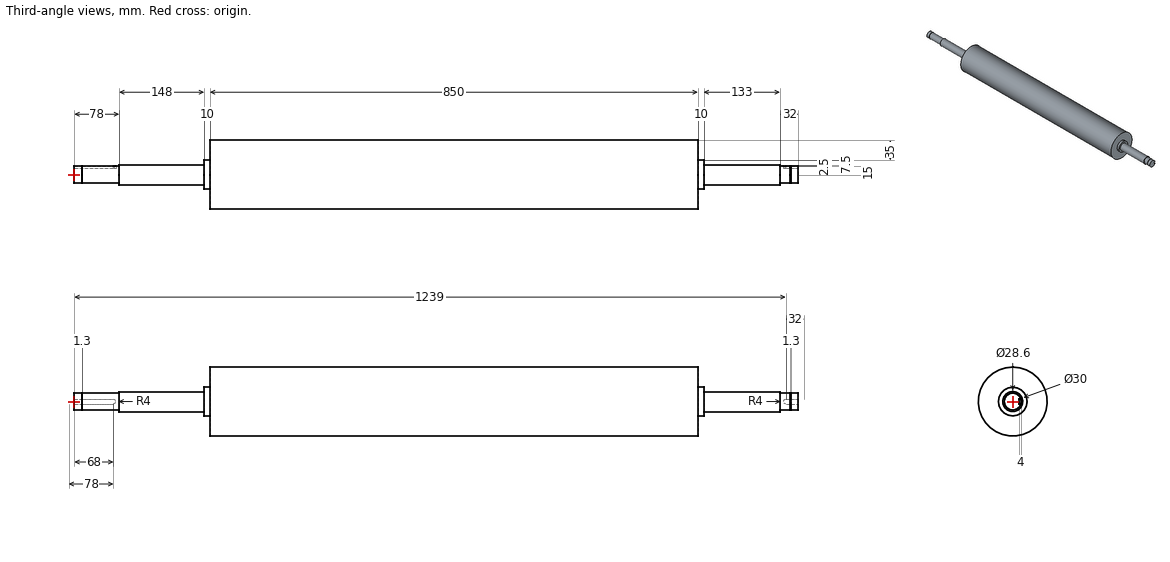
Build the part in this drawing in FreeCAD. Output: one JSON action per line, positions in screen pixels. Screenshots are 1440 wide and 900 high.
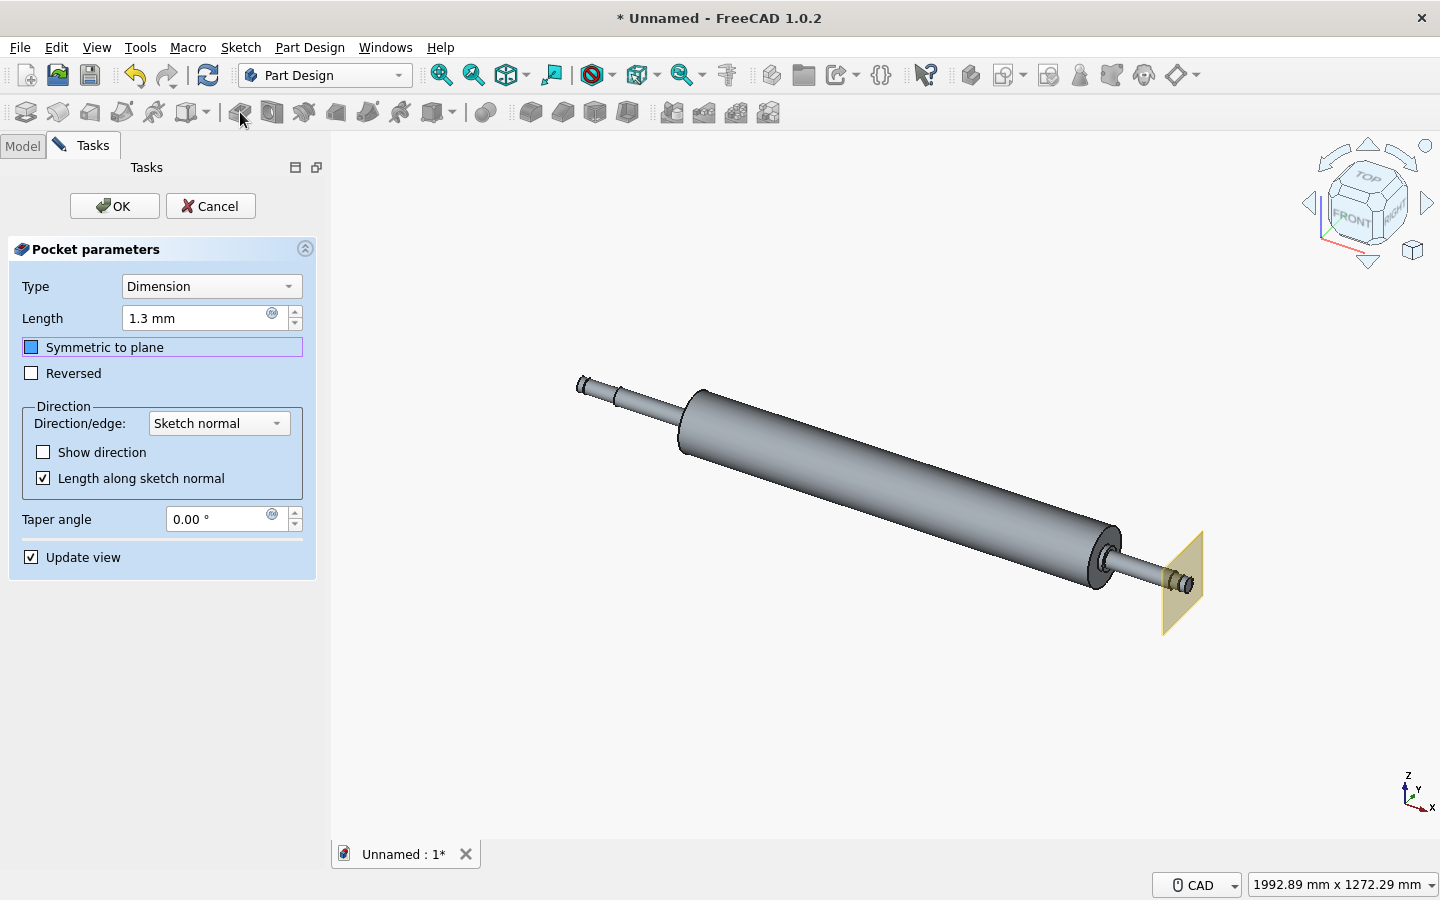
{"action": "left_click", "coordinate": [115, 206]}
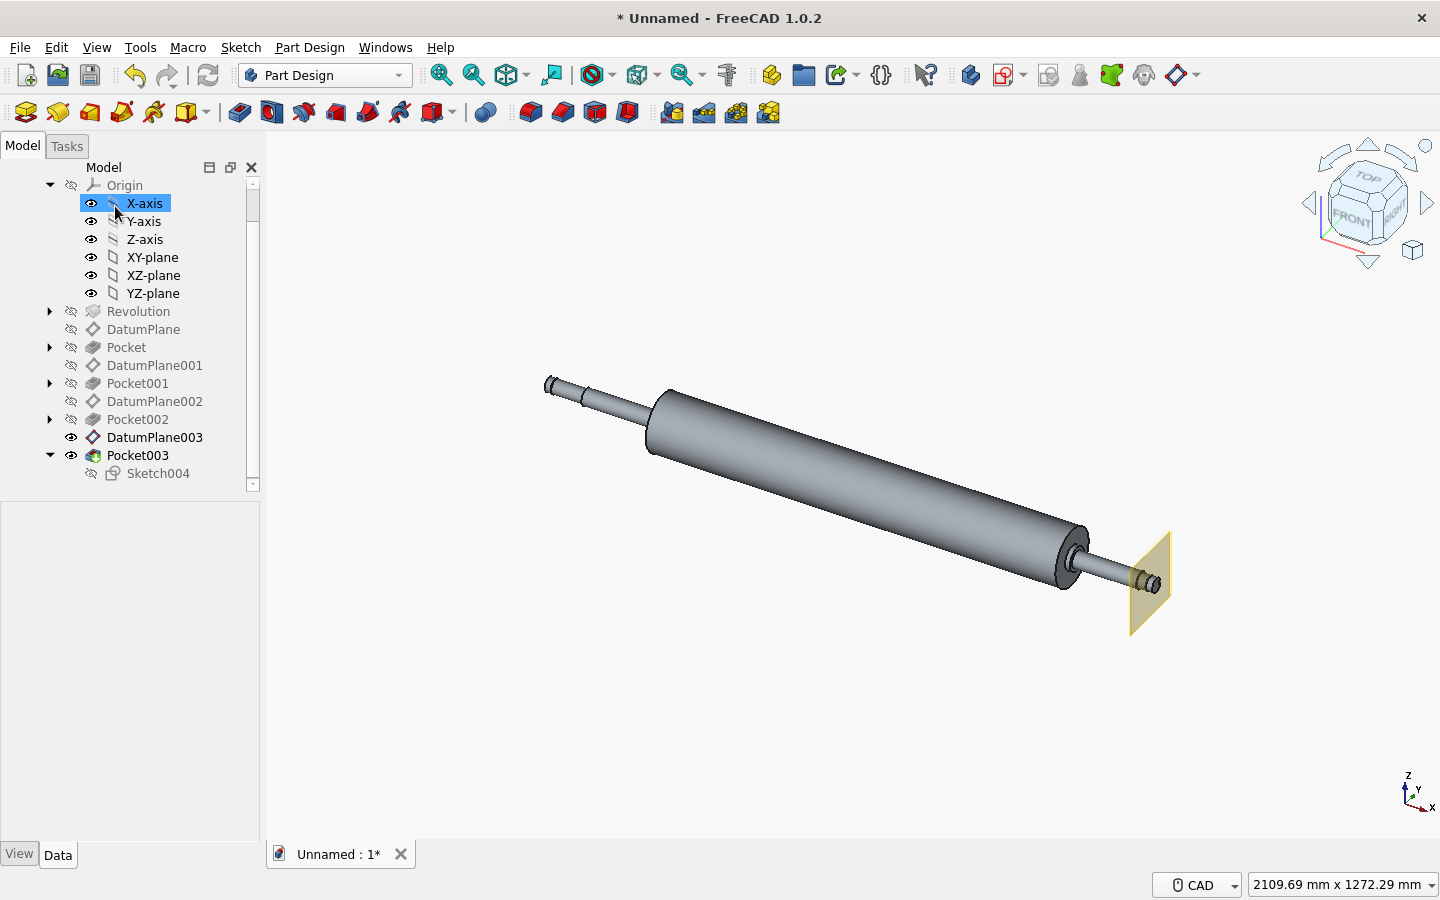
{"action": "left_click", "coordinate": [116, 437]}
{"action": "key", "text": "space"}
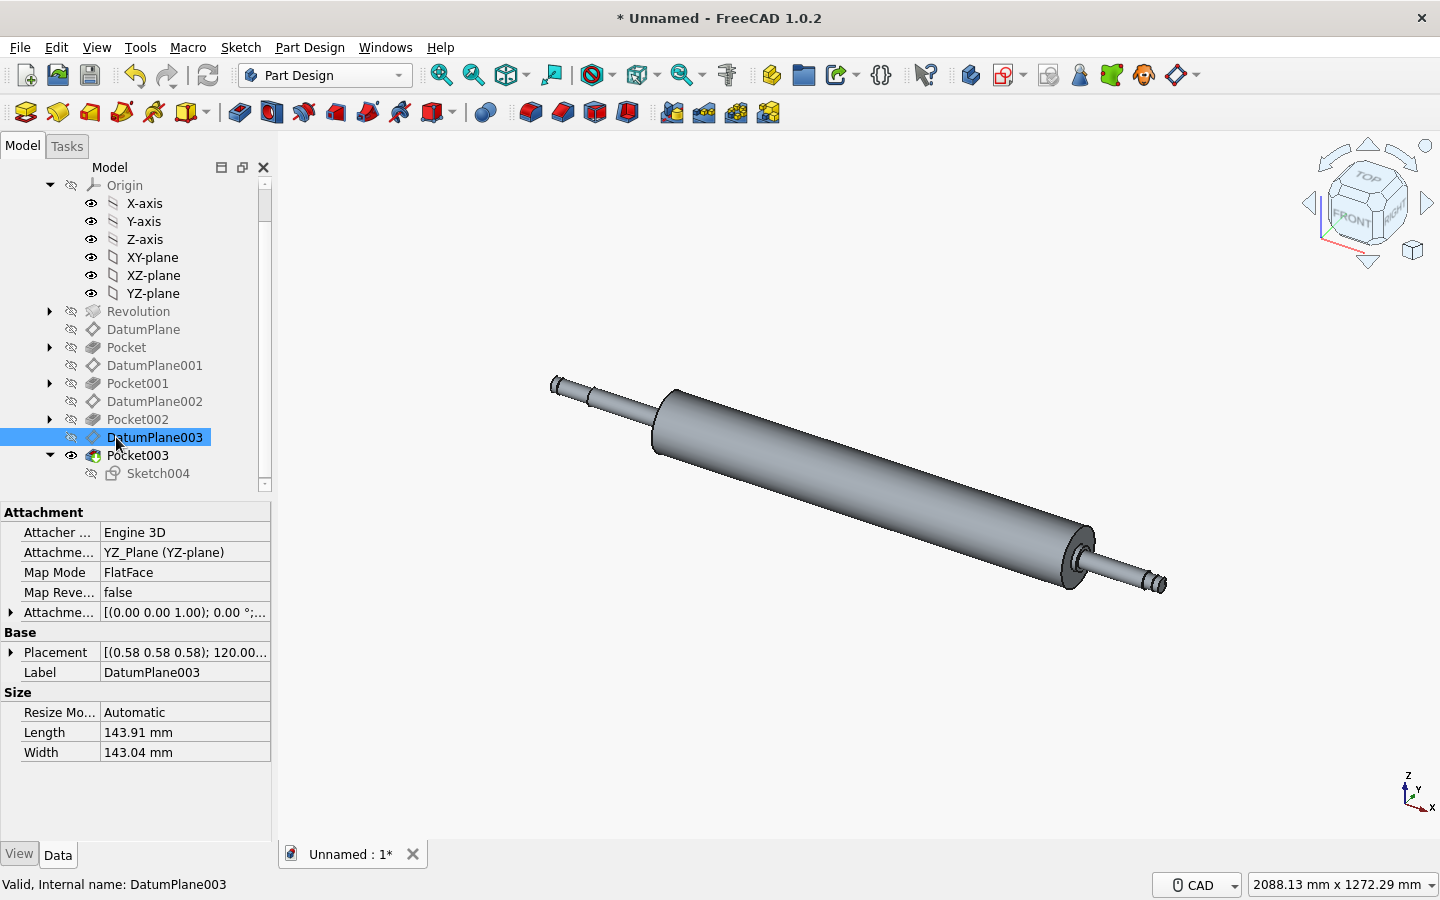
{"action": "key", "text": "0"}